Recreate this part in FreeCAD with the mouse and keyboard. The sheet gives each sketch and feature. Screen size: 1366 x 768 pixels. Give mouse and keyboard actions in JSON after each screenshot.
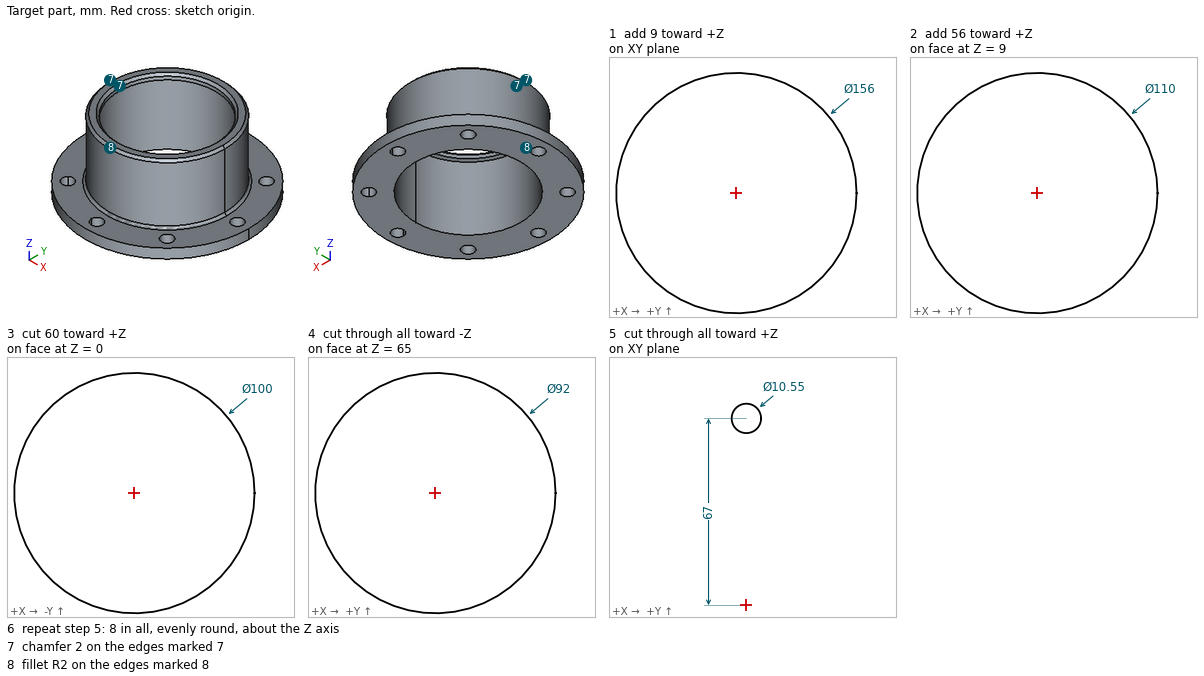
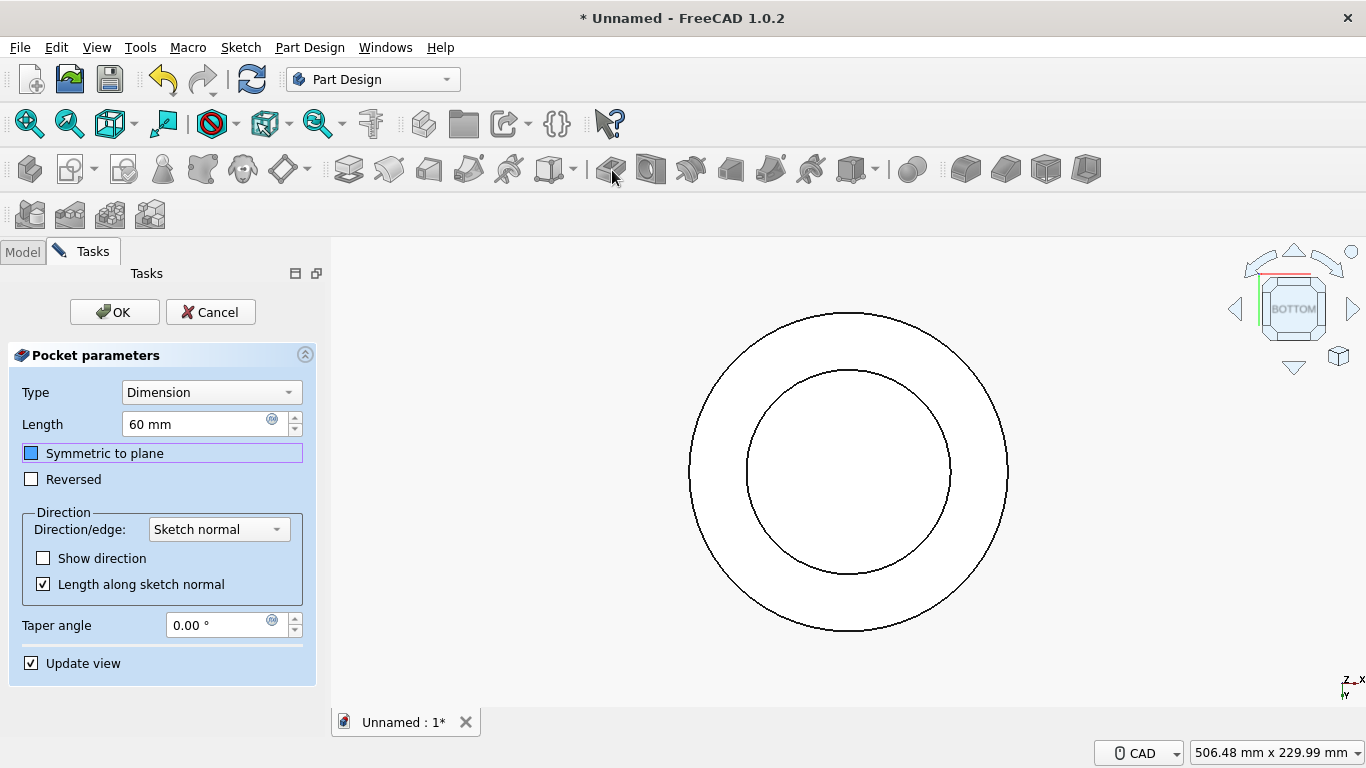
{"action": "left_click", "coordinate": [115, 312]}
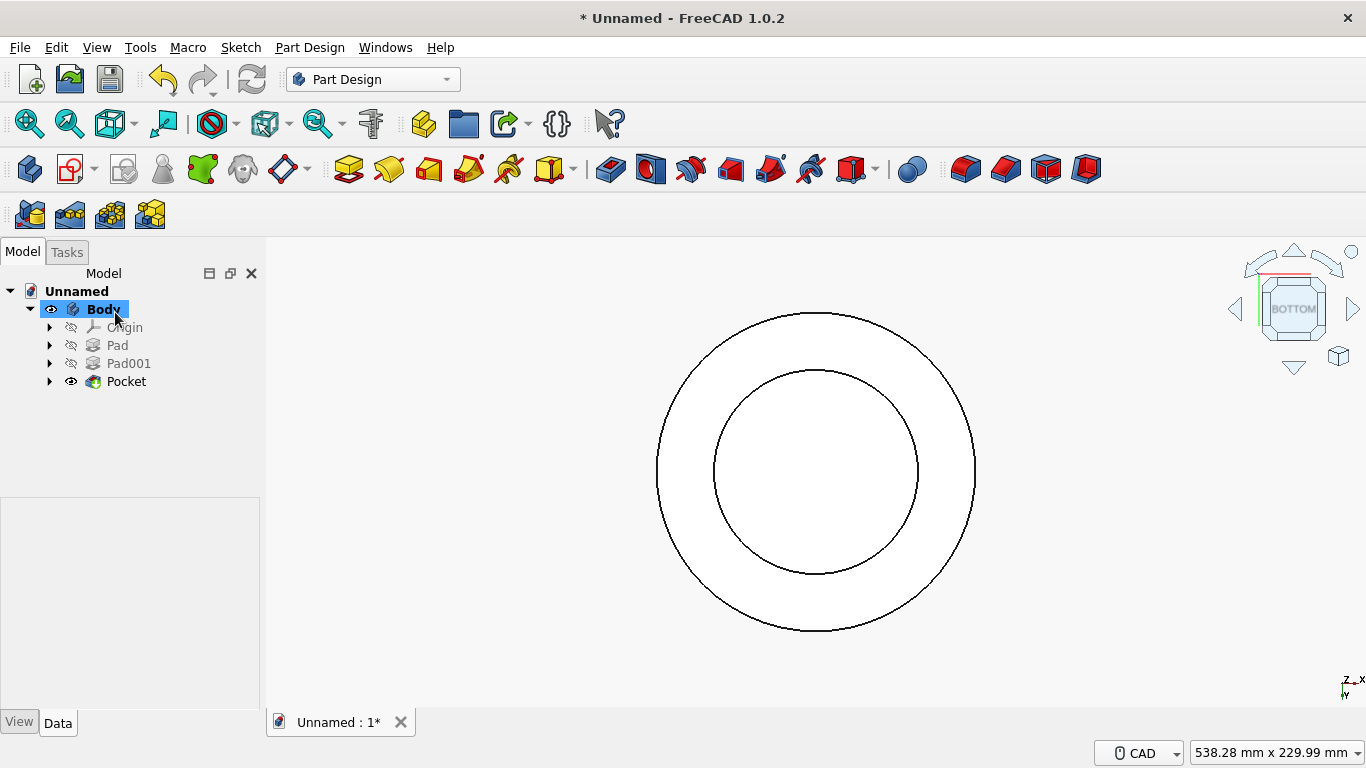
{"action": "key", "text": "0"}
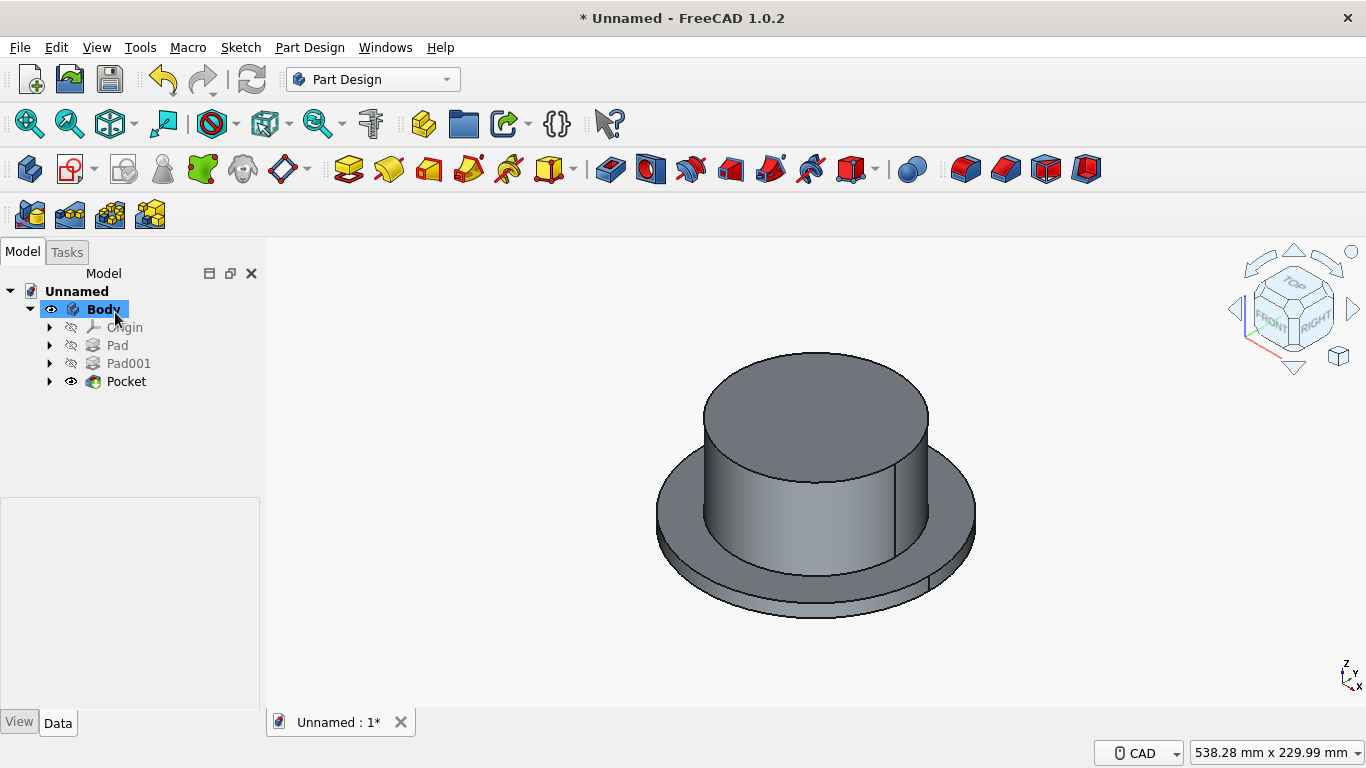
{"action": "left_click", "coordinate": [816, 417]}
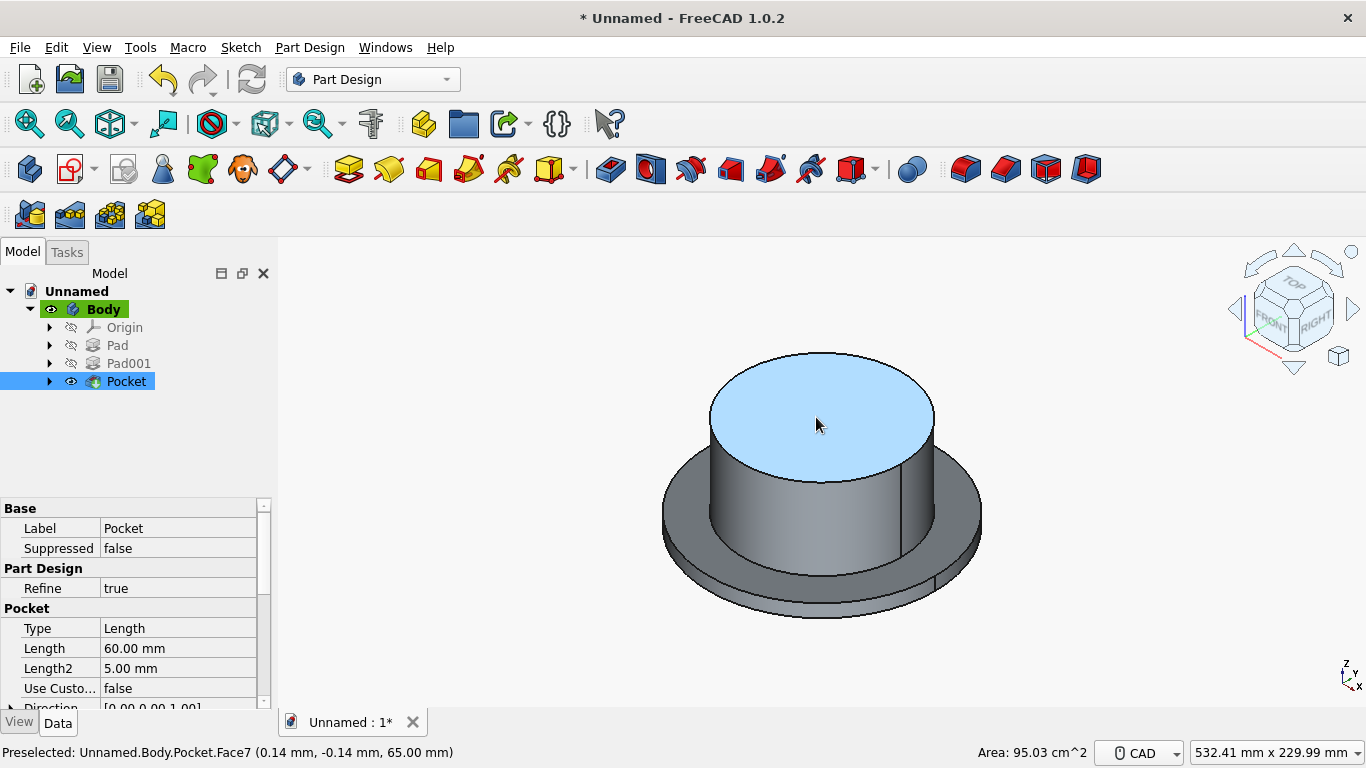
{"action": "left_click", "coordinate": [70, 170]}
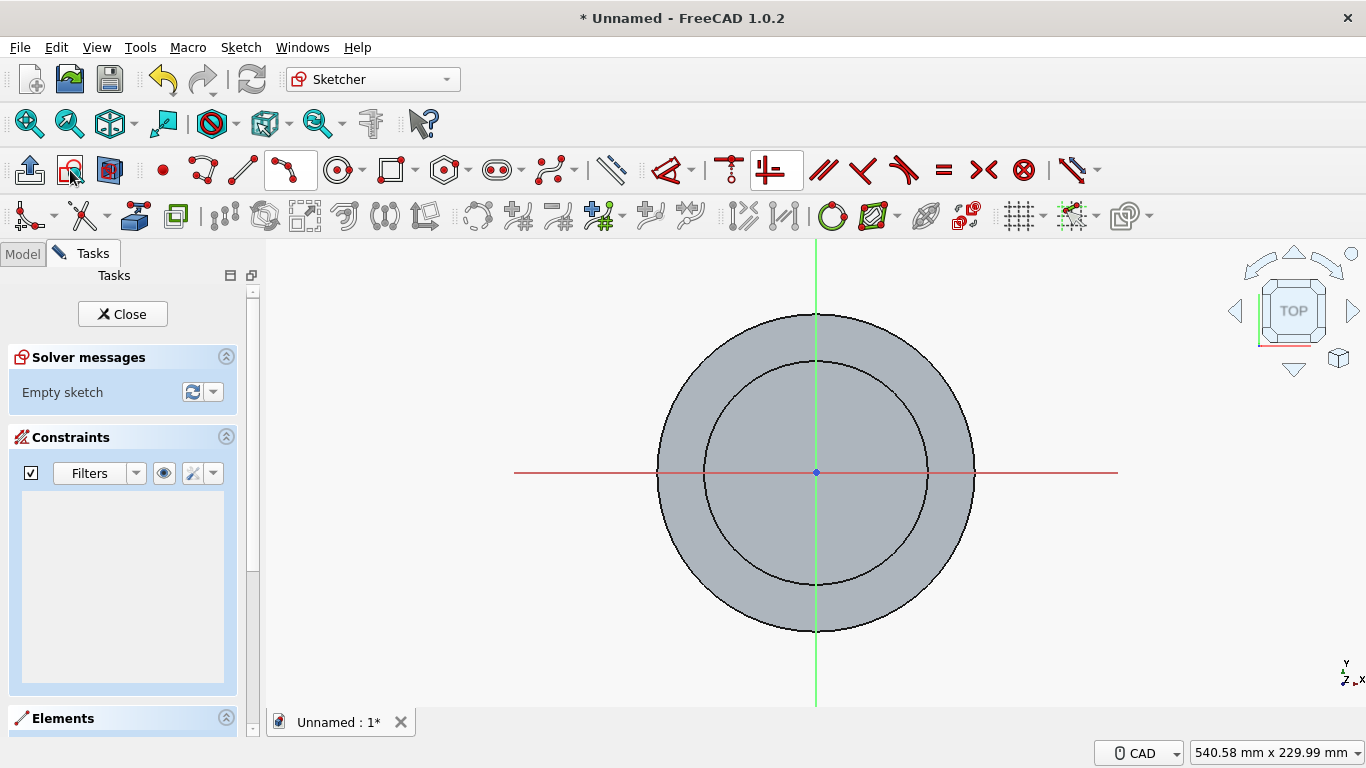
{"action": "scroll", "coordinate": [955, 473], "scroll_direction": "up", "scroll_amount": 2}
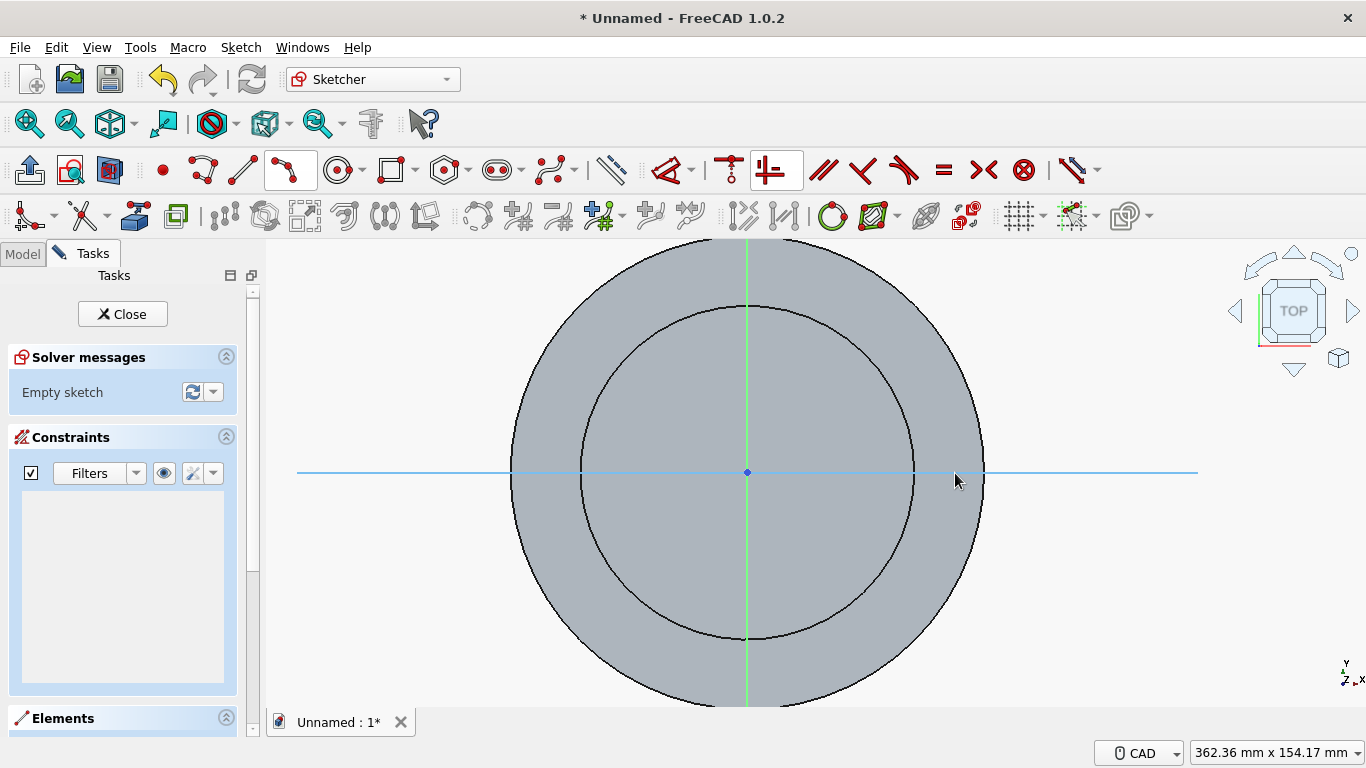
{"action": "key", "text": "g c"}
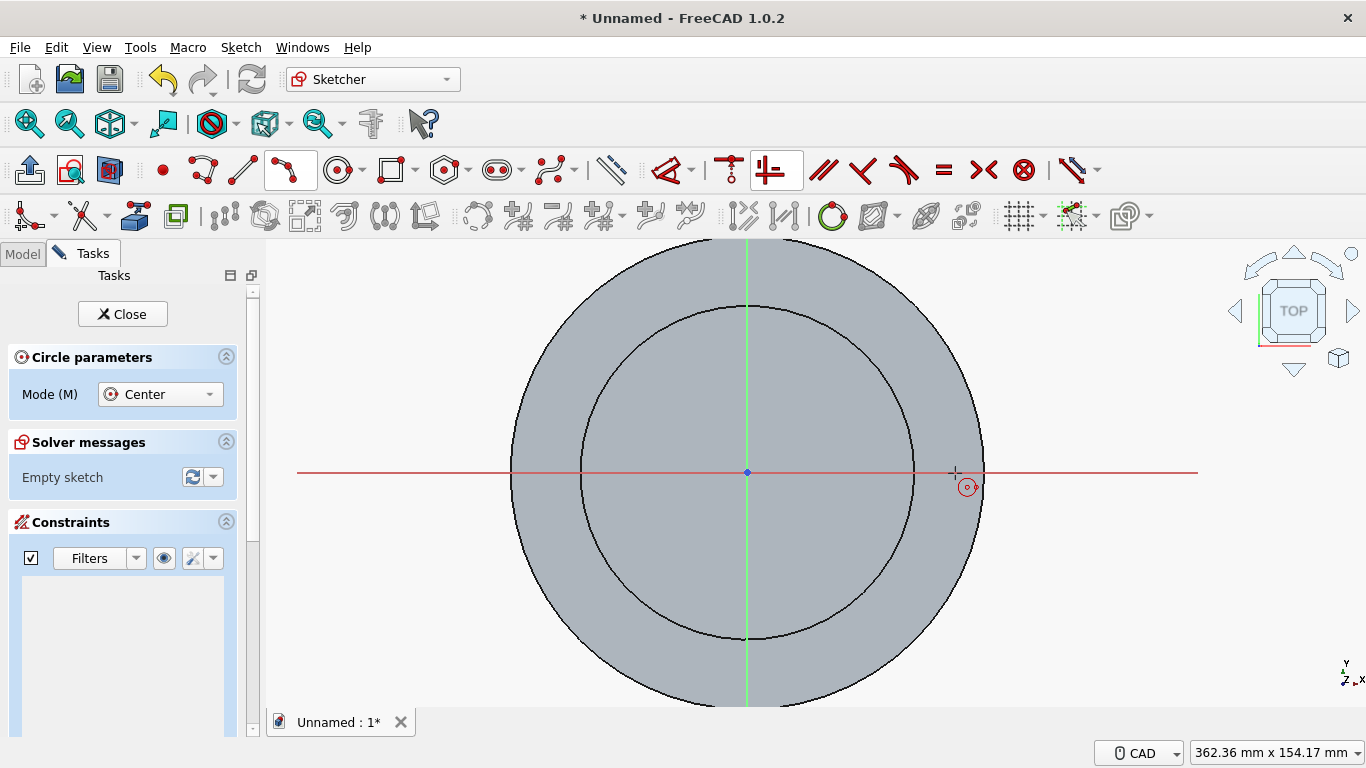
{"action": "left_click", "coordinate": [747, 473]}
{"action": "left_click", "coordinate": [846, 374]}
{"action": "key", "text": "Escape"}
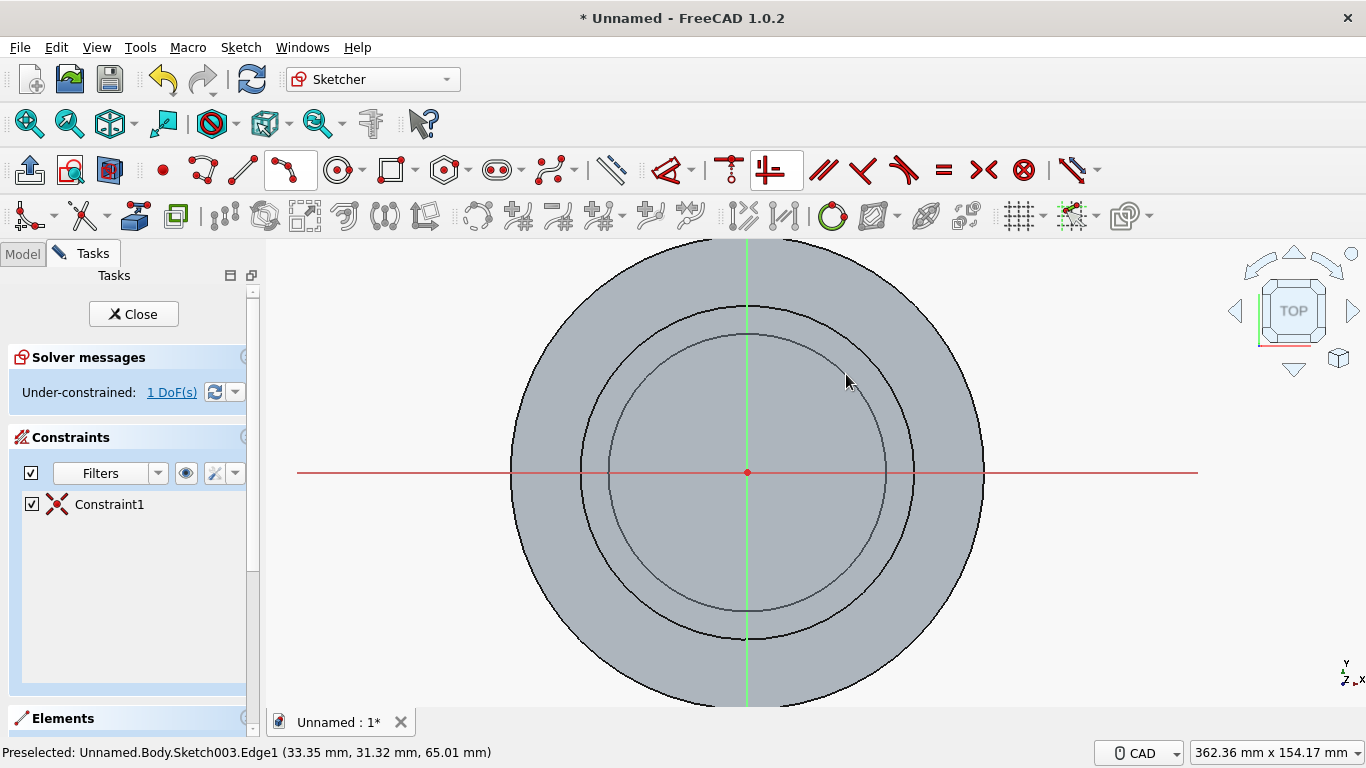
{"action": "left_click", "coordinate": [666, 170]}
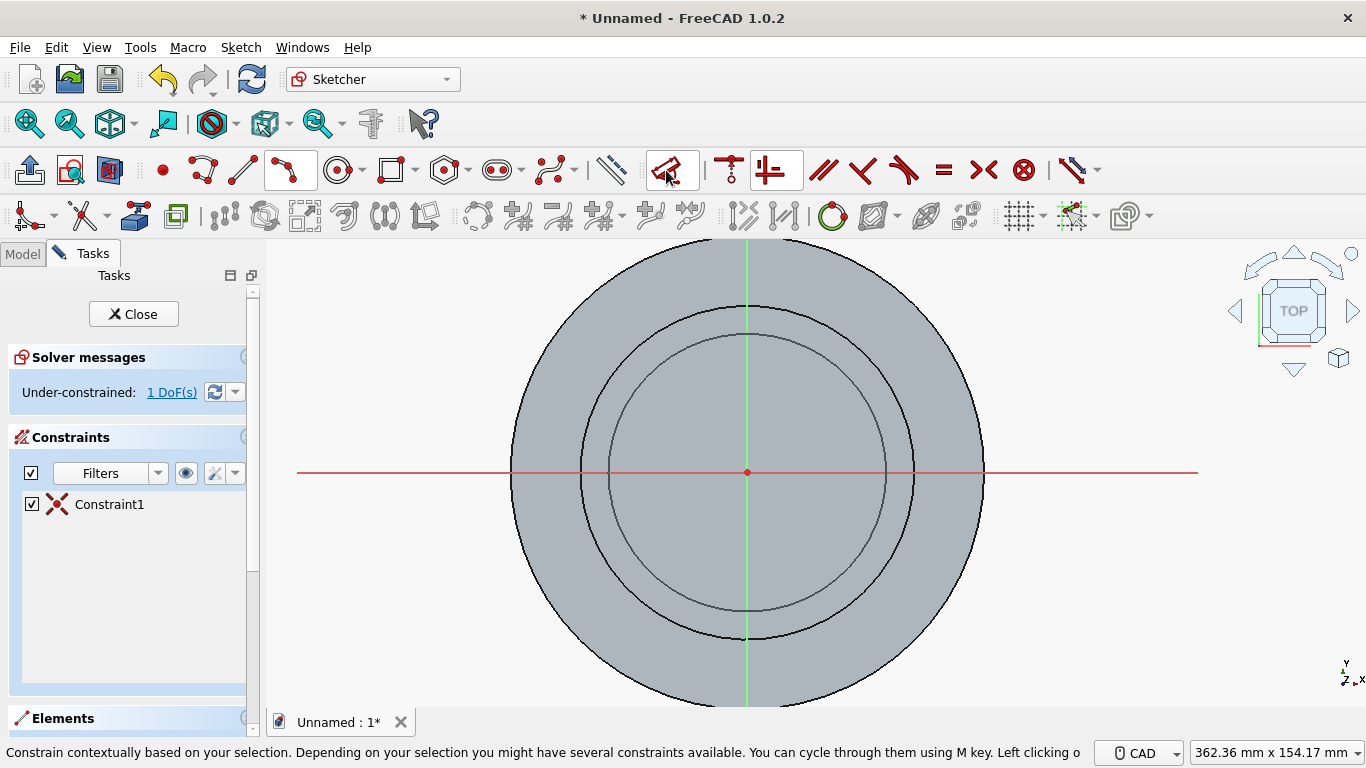
{"action": "left_click", "coordinate": [845, 374]}
{"action": "left_click", "coordinate": [868, 351]}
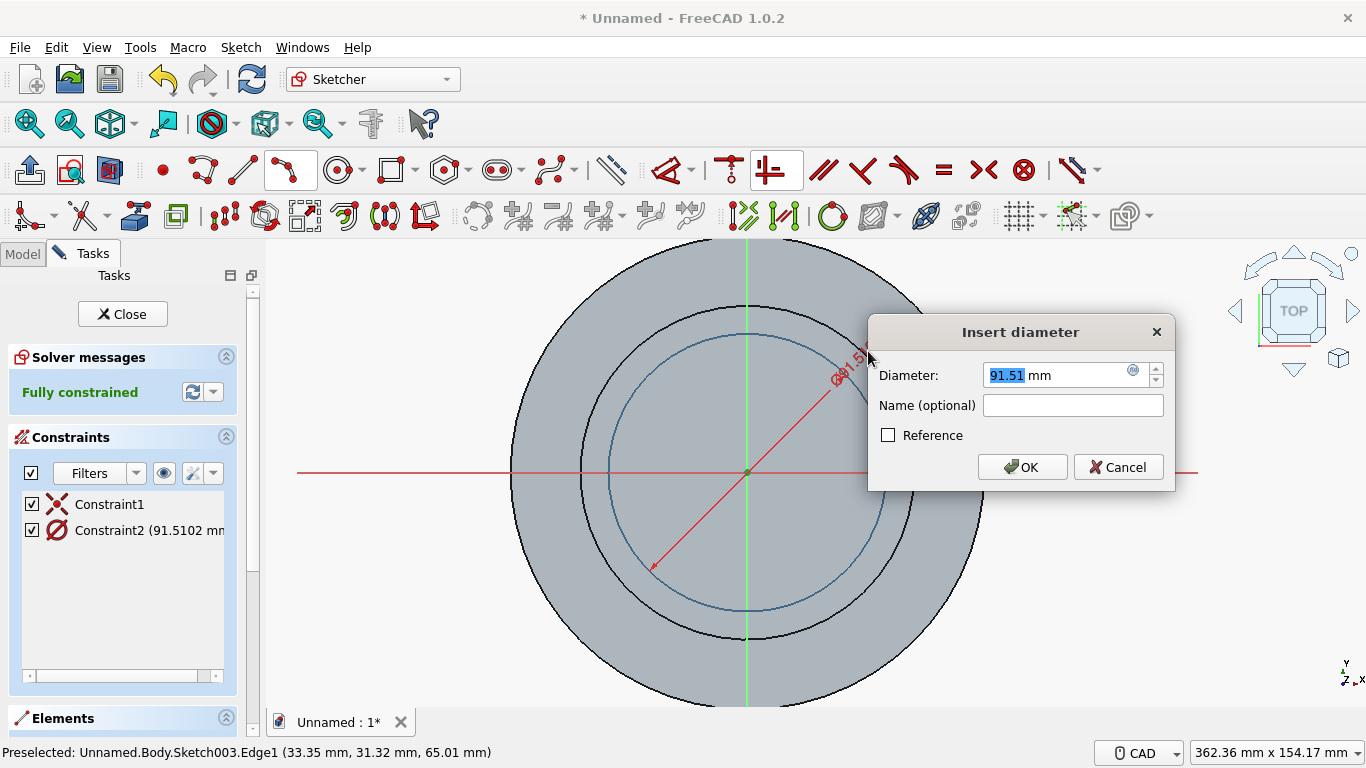
{"action": "type", "text": "92"}
{"action": "key", "text": "Return"}
{"action": "key", "text": "Escape"}